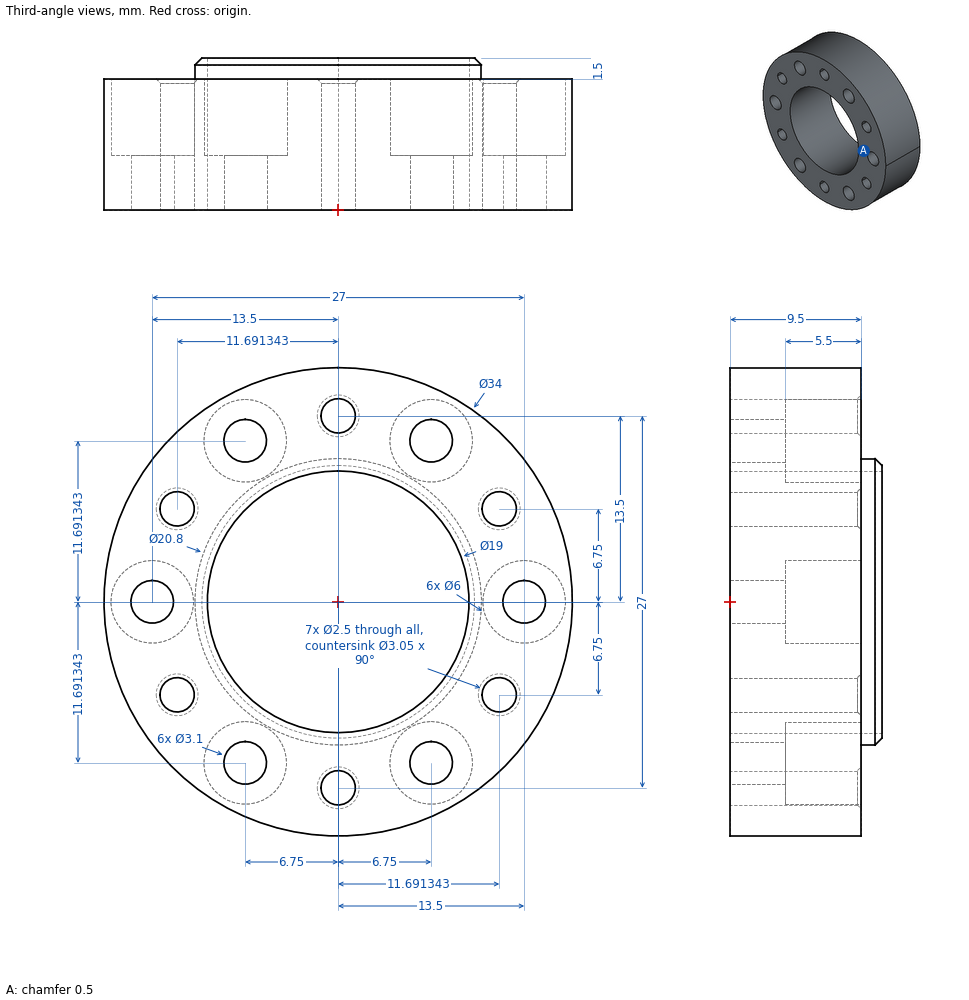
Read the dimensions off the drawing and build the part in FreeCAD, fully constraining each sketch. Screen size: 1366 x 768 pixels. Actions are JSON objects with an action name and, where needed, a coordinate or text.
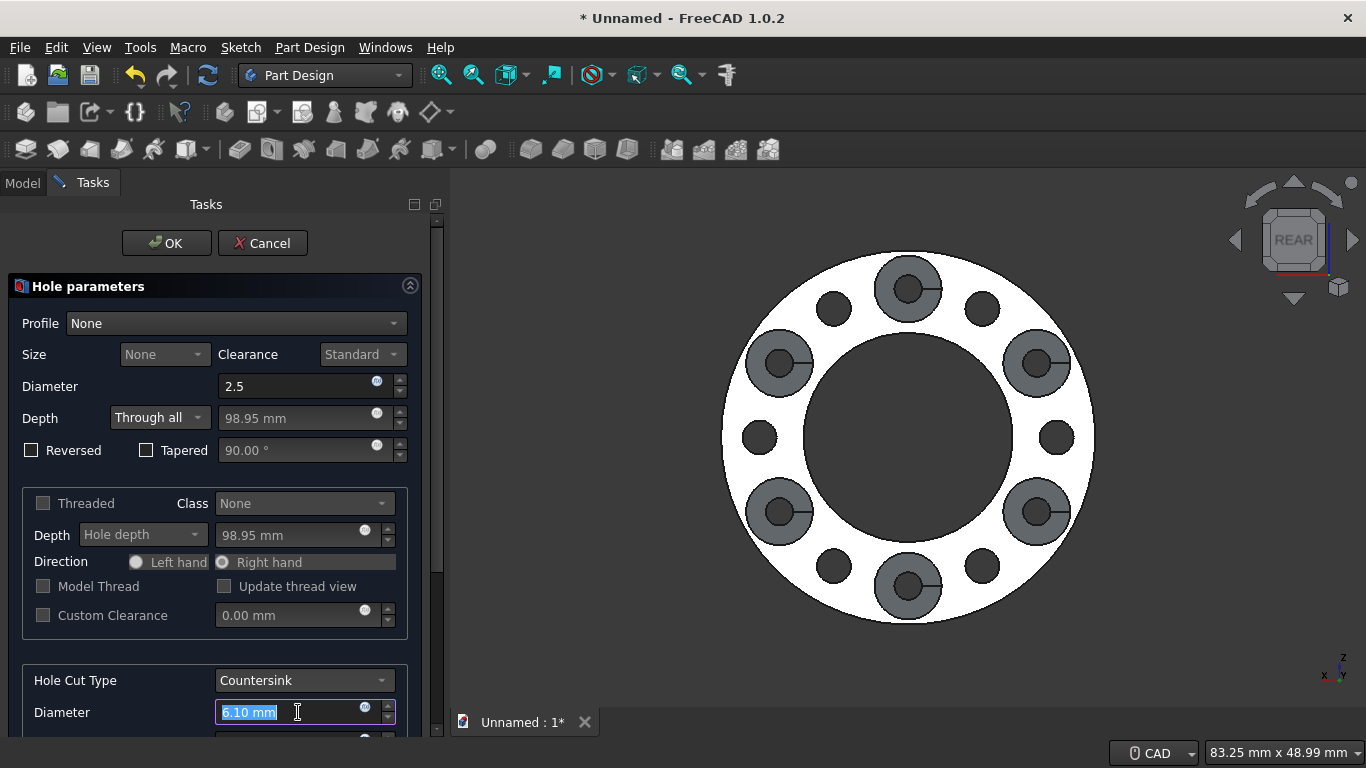
{"action": "type", "text": "3.05"}
{"action": "key", "text": "Tab"}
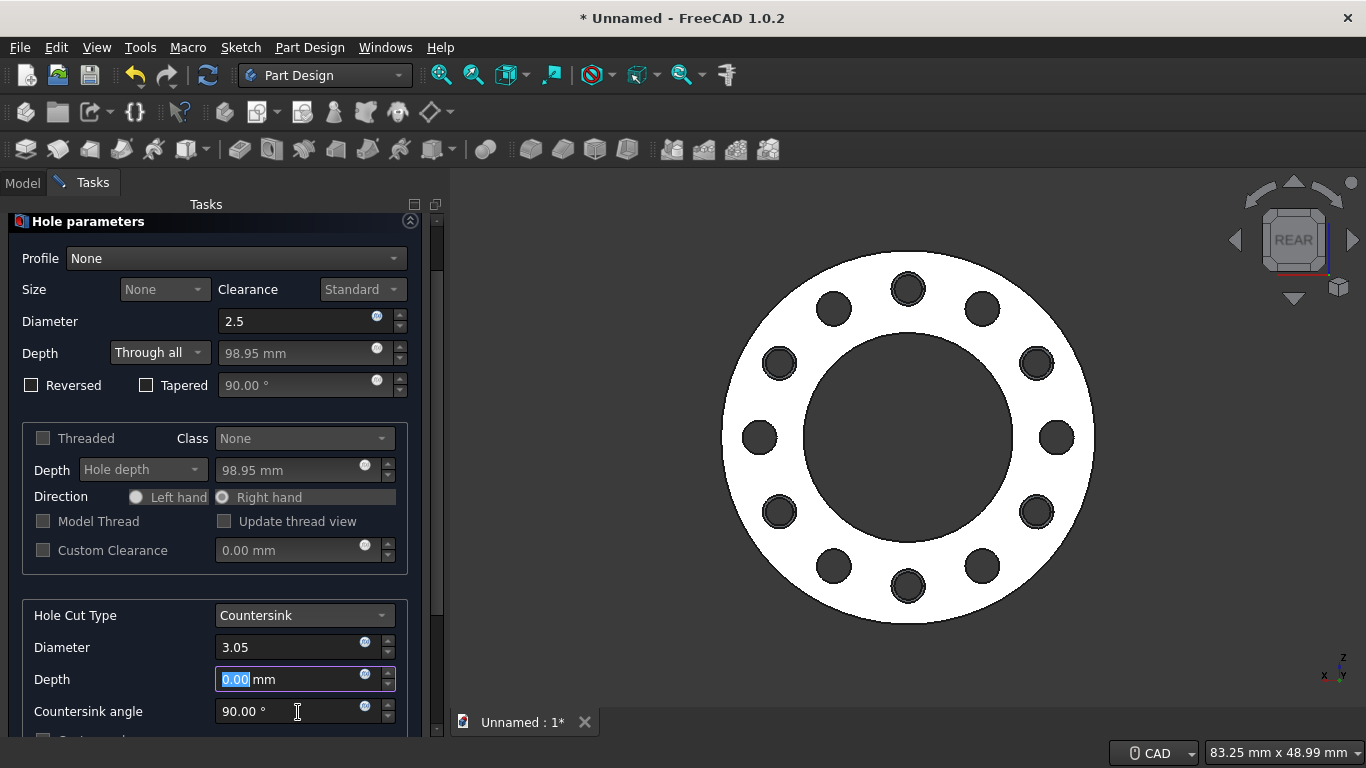
{"action": "scroll", "coordinate": [437, 475], "scroll_direction": "up", "scroll_amount": 2}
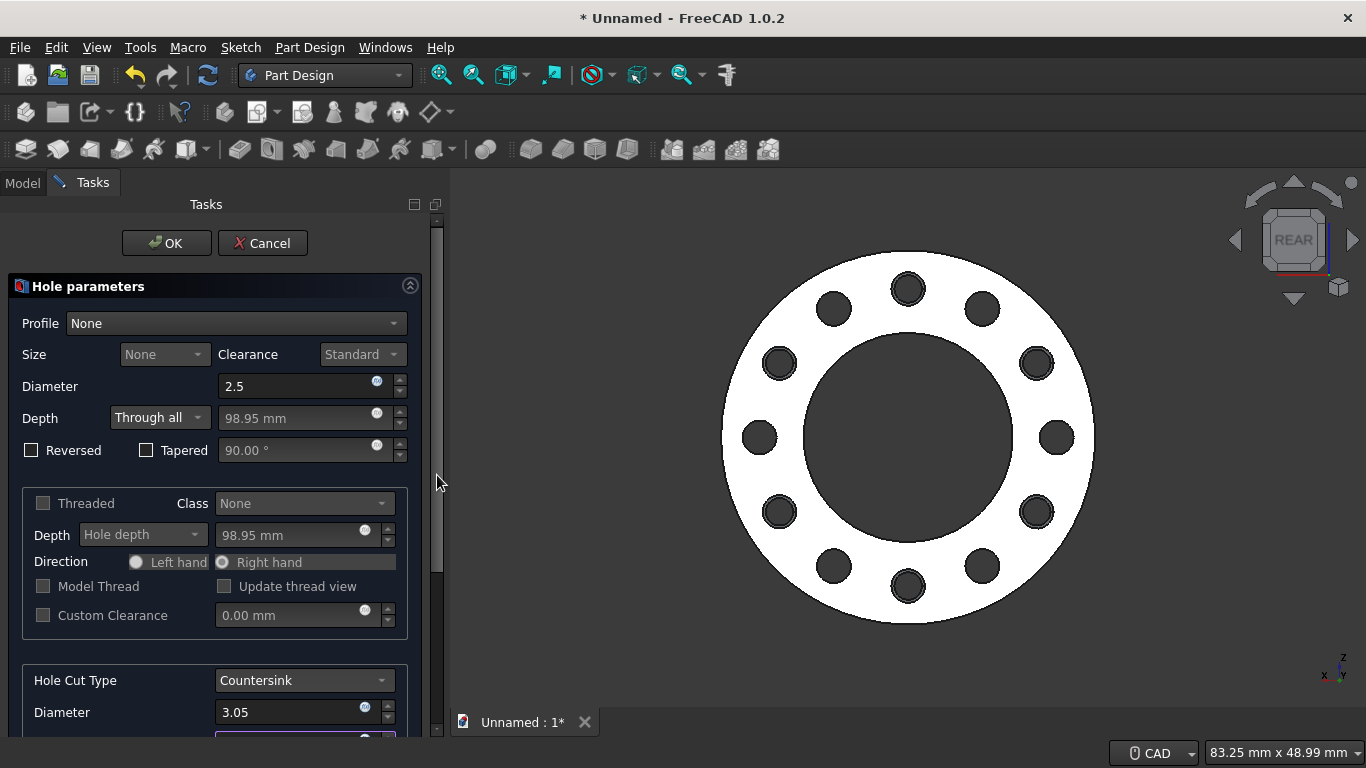
{"action": "left_click", "coordinate": [167, 243]}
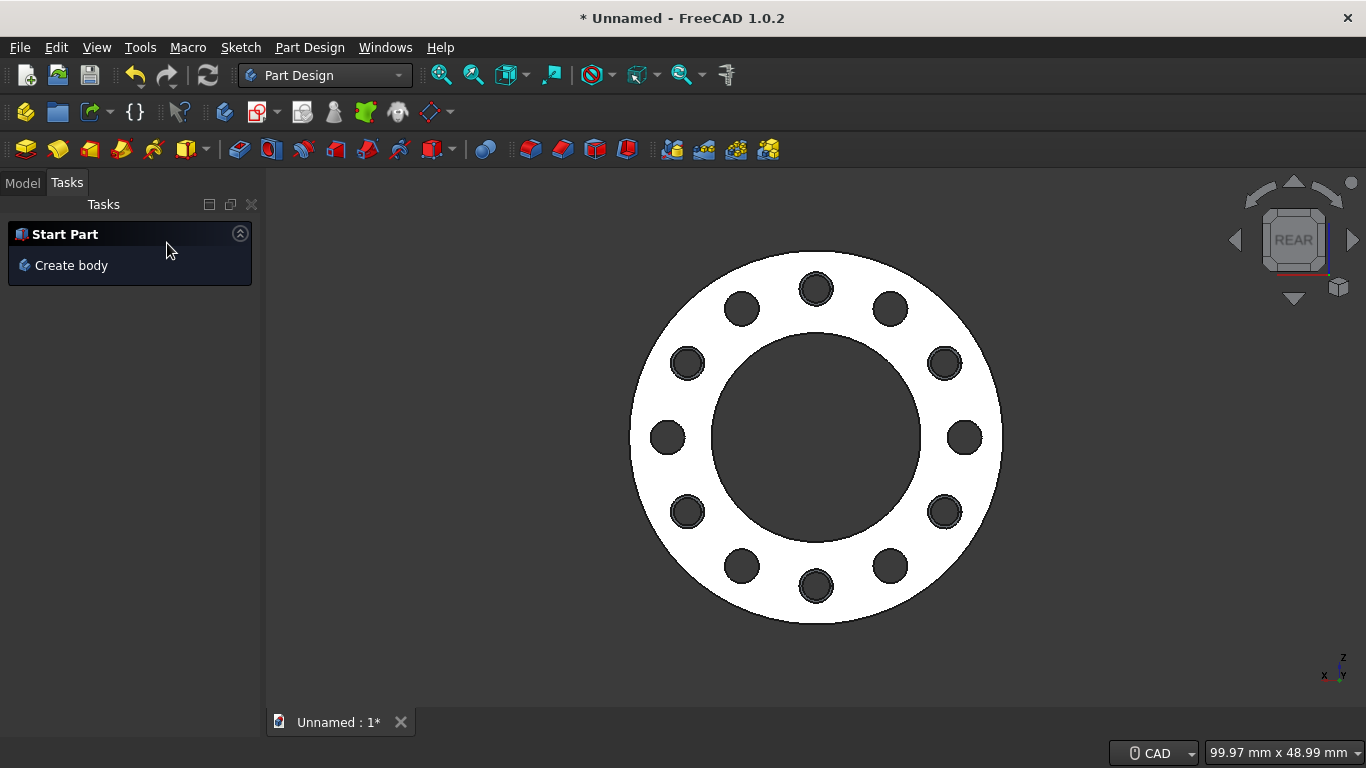
{"action": "left_click", "coordinate": [709, 330]}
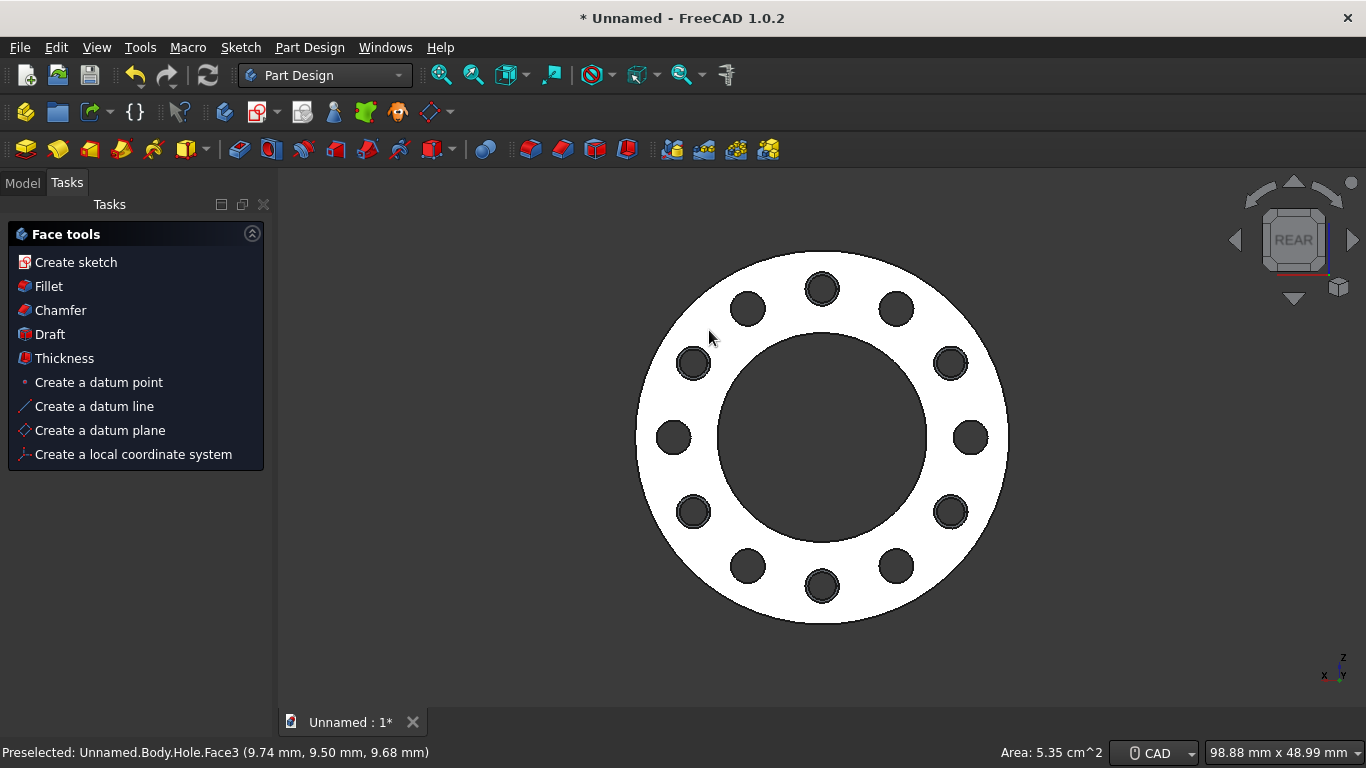
{"action": "left_click", "coordinate": [258, 112]}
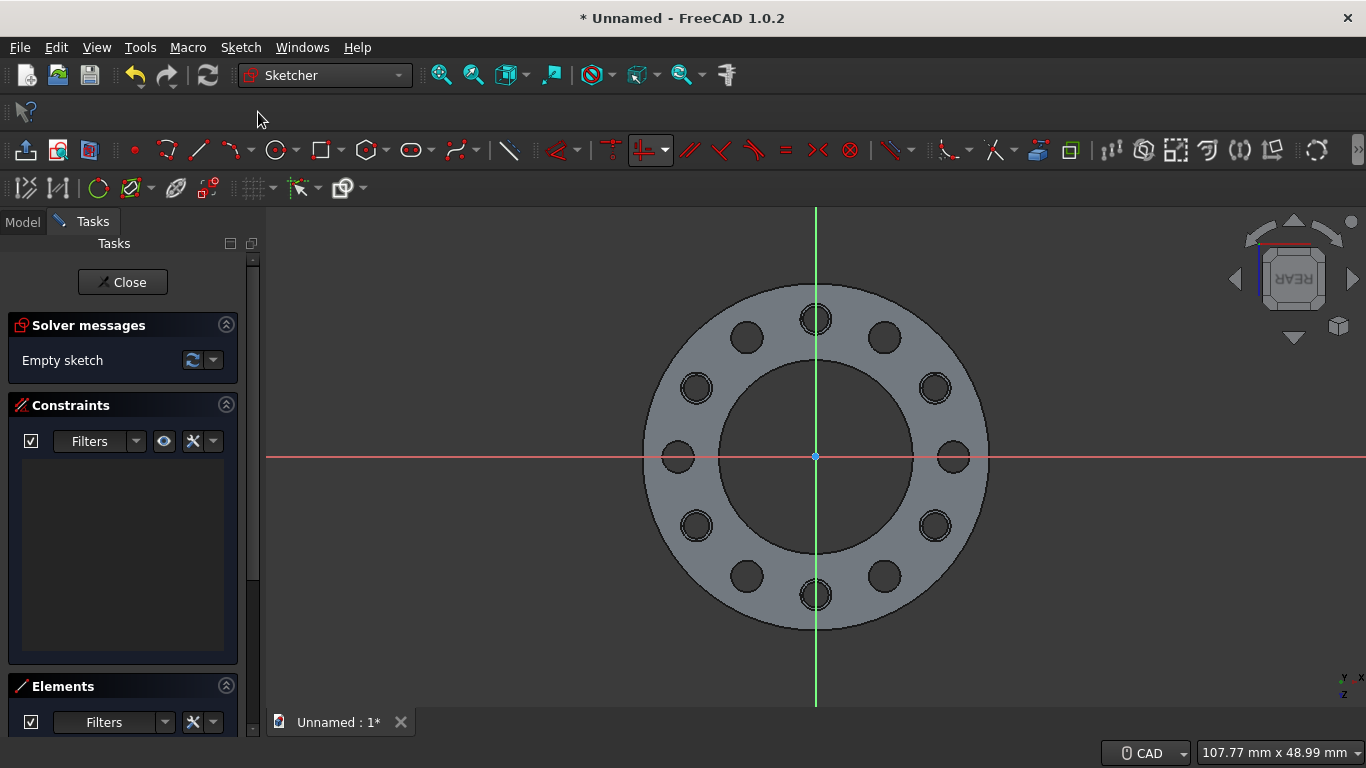
{"action": "scroll", "coordinate": [955, 457], "scroll_direction": "up", "scroll_amount": 2}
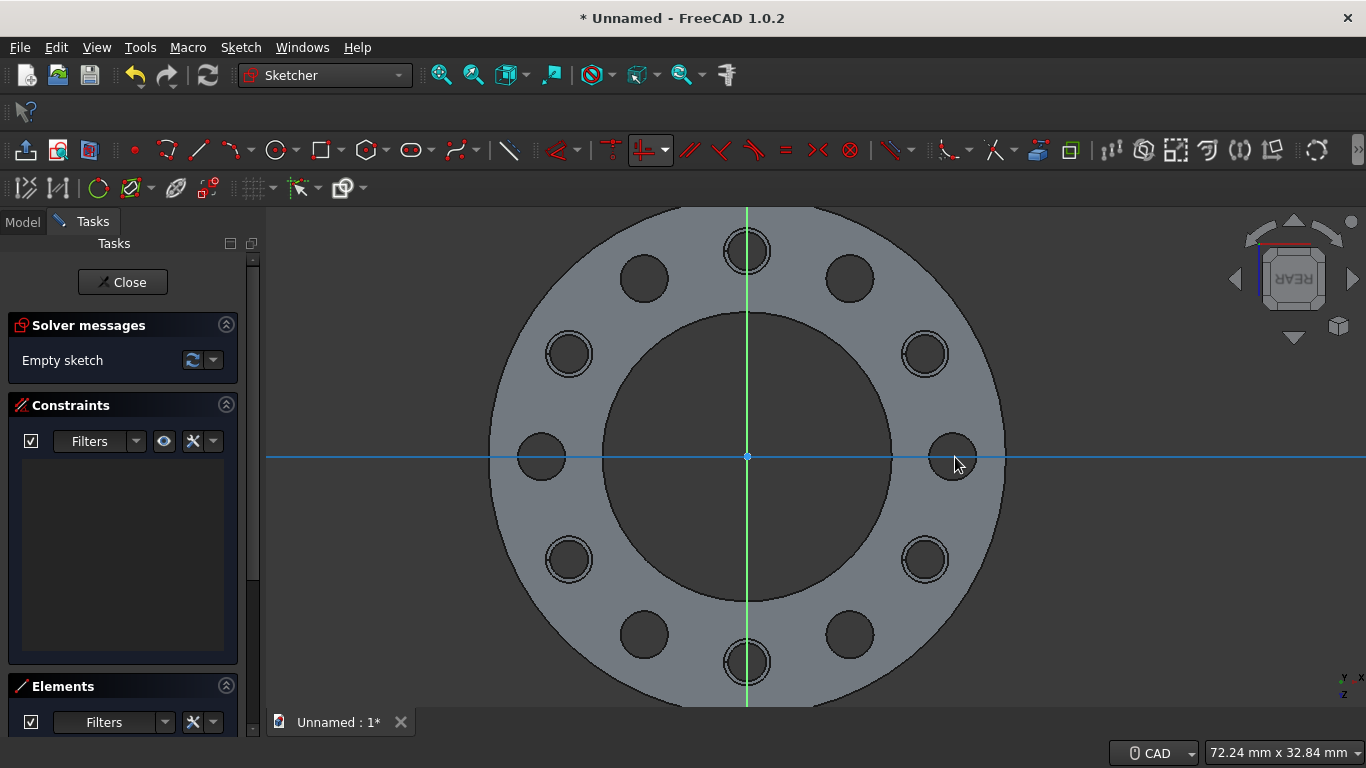
{"action": "left_click", "coordinate": [276, 150]}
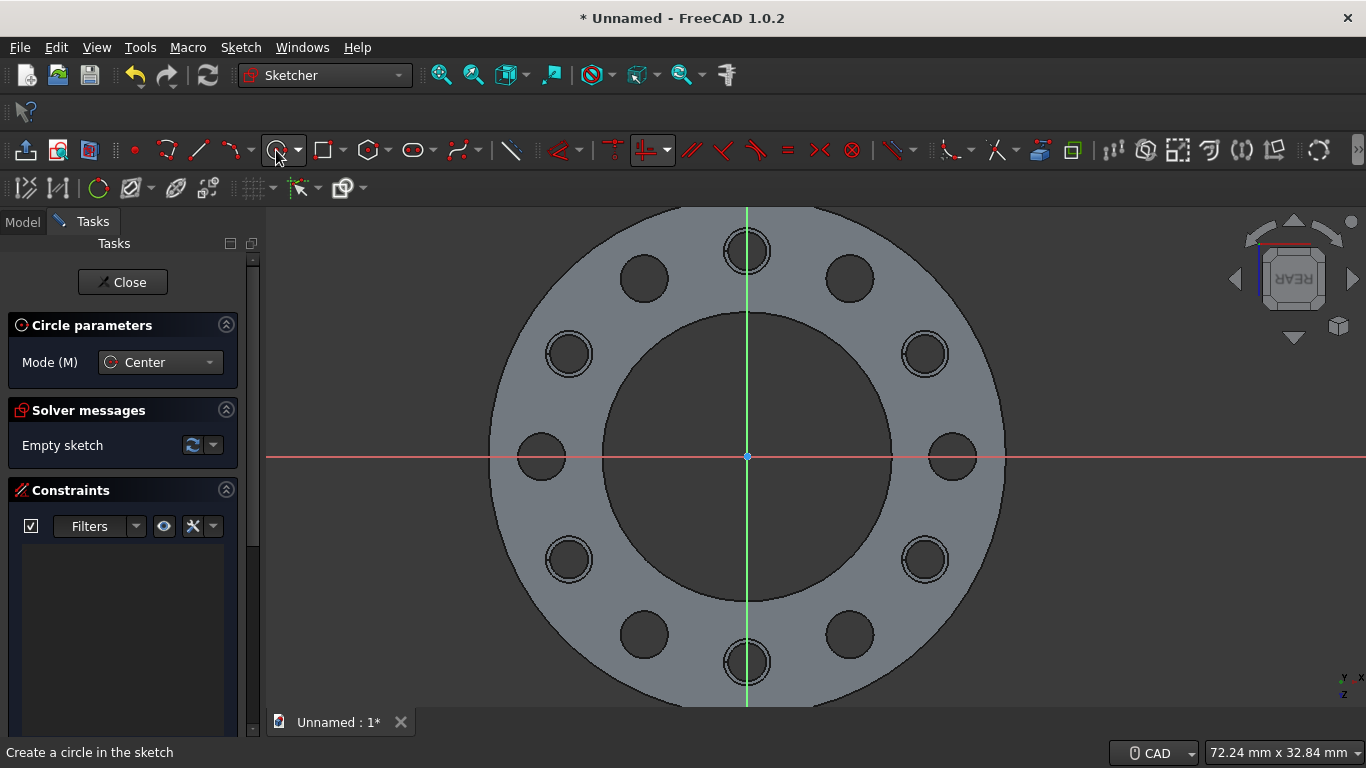
{"action": "left_click", "coordinate": [747, 457]}
{"action": "mouse_move", "coordinate": [859, 345]}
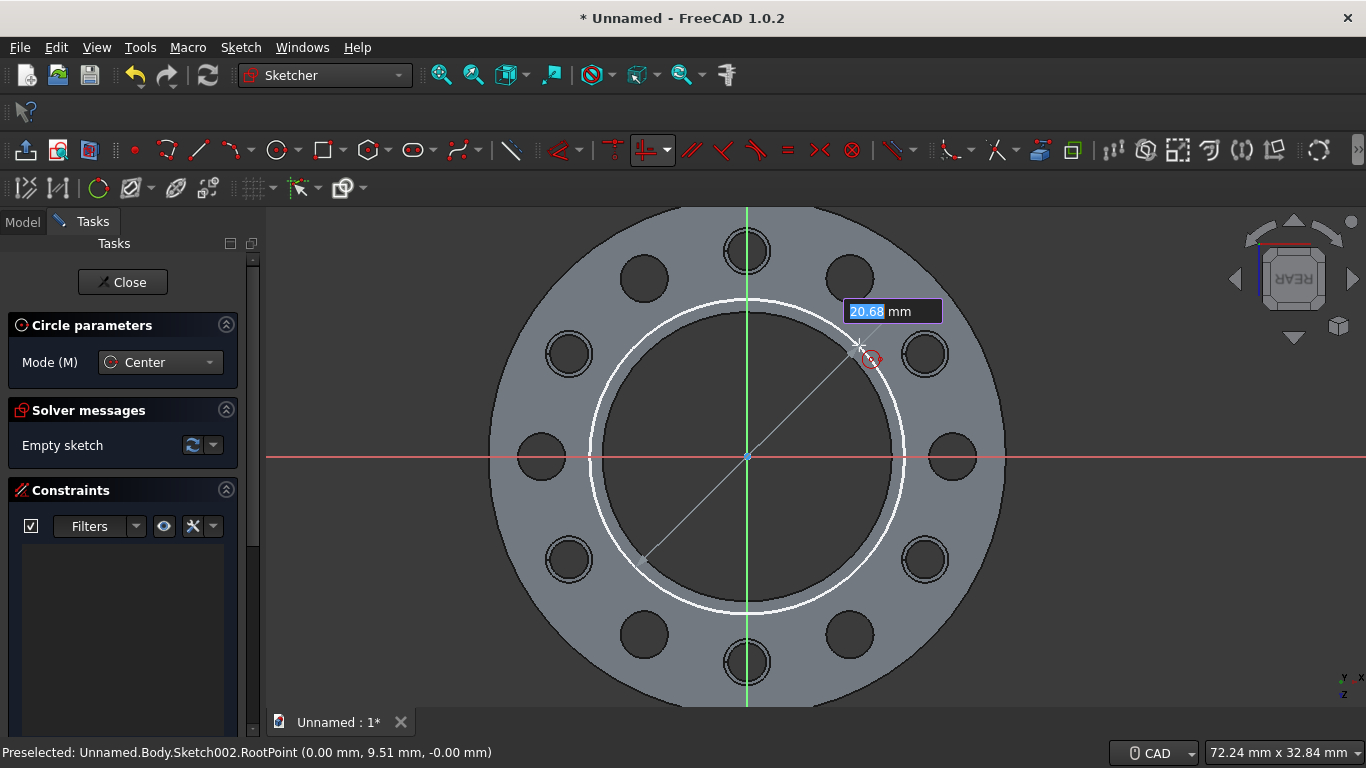
{"action": "type", "text": "20.8"}
{"action": "key", "text": "Return"}